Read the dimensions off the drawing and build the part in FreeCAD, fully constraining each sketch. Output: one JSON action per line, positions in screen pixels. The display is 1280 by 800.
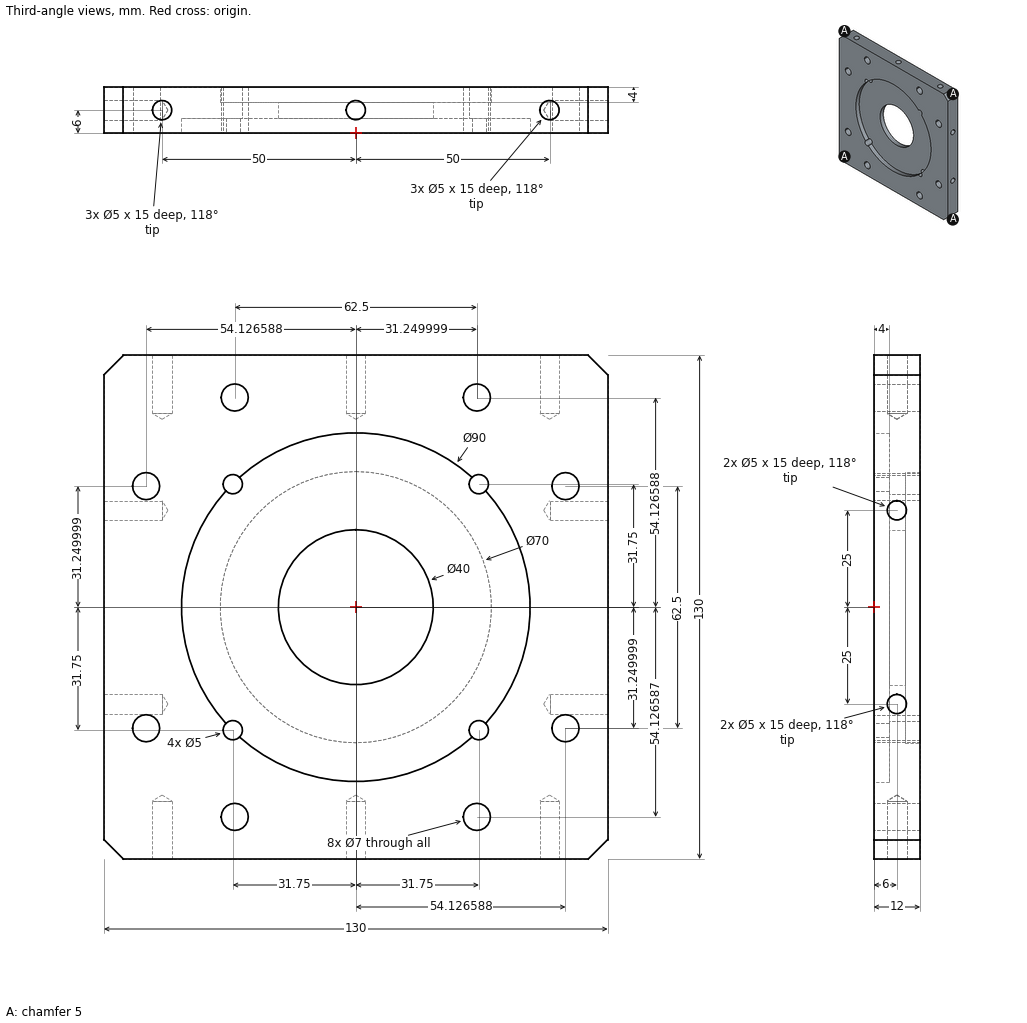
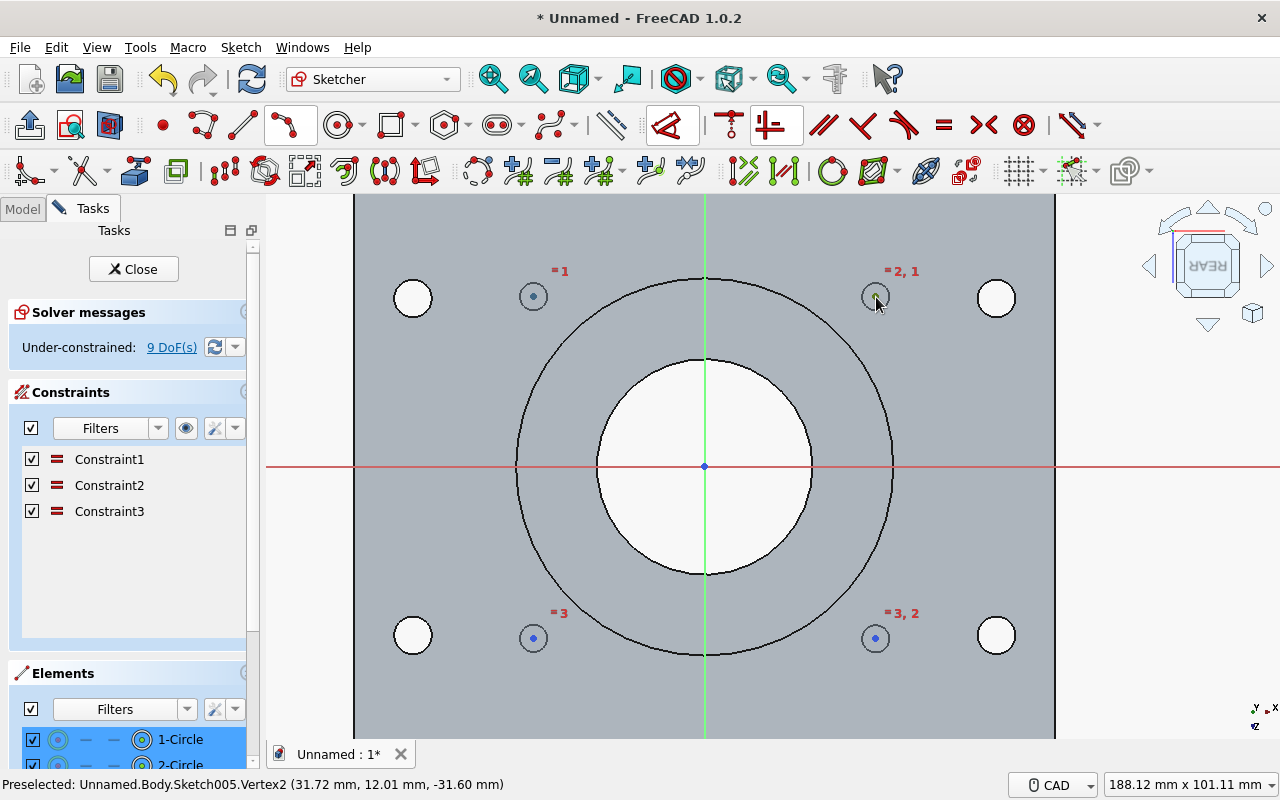
{"action": "left_click", "coordinate": [798, 126]}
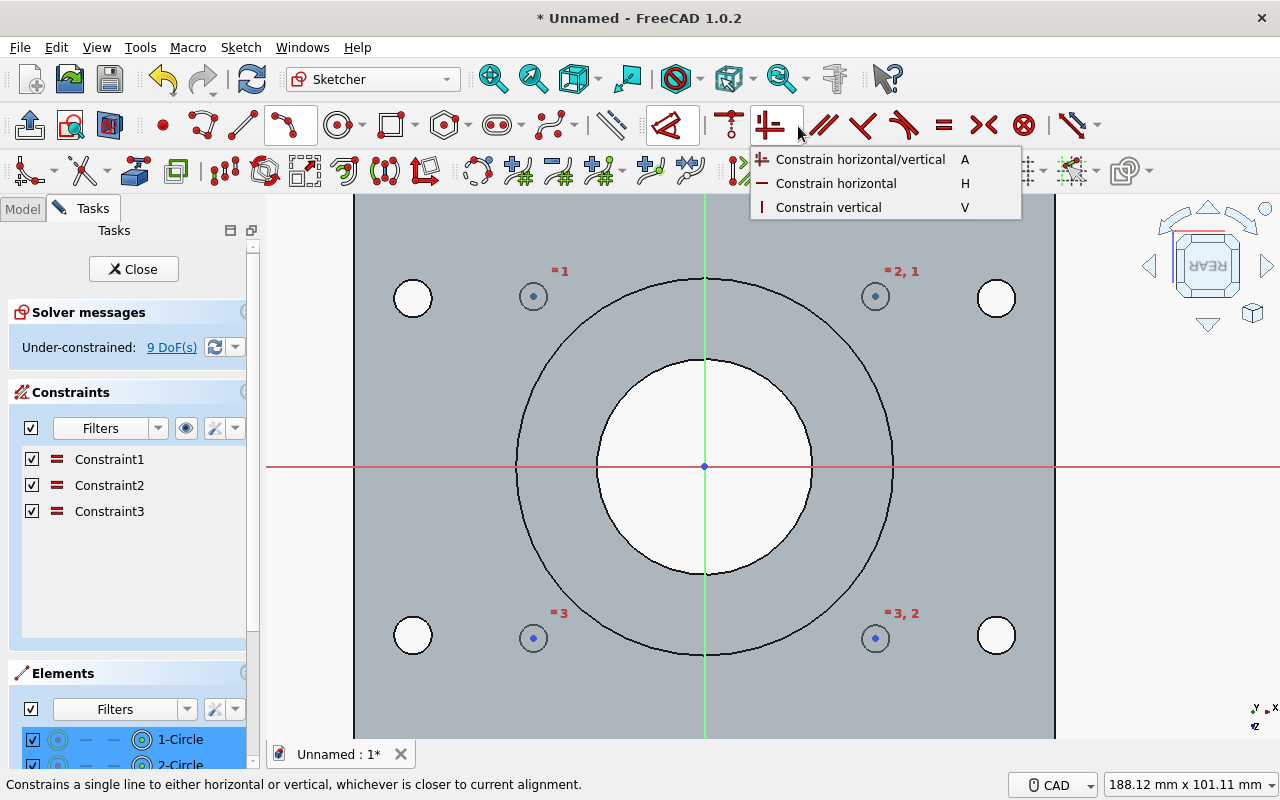
{"action": "left_click", "coordinate": [886, 183]}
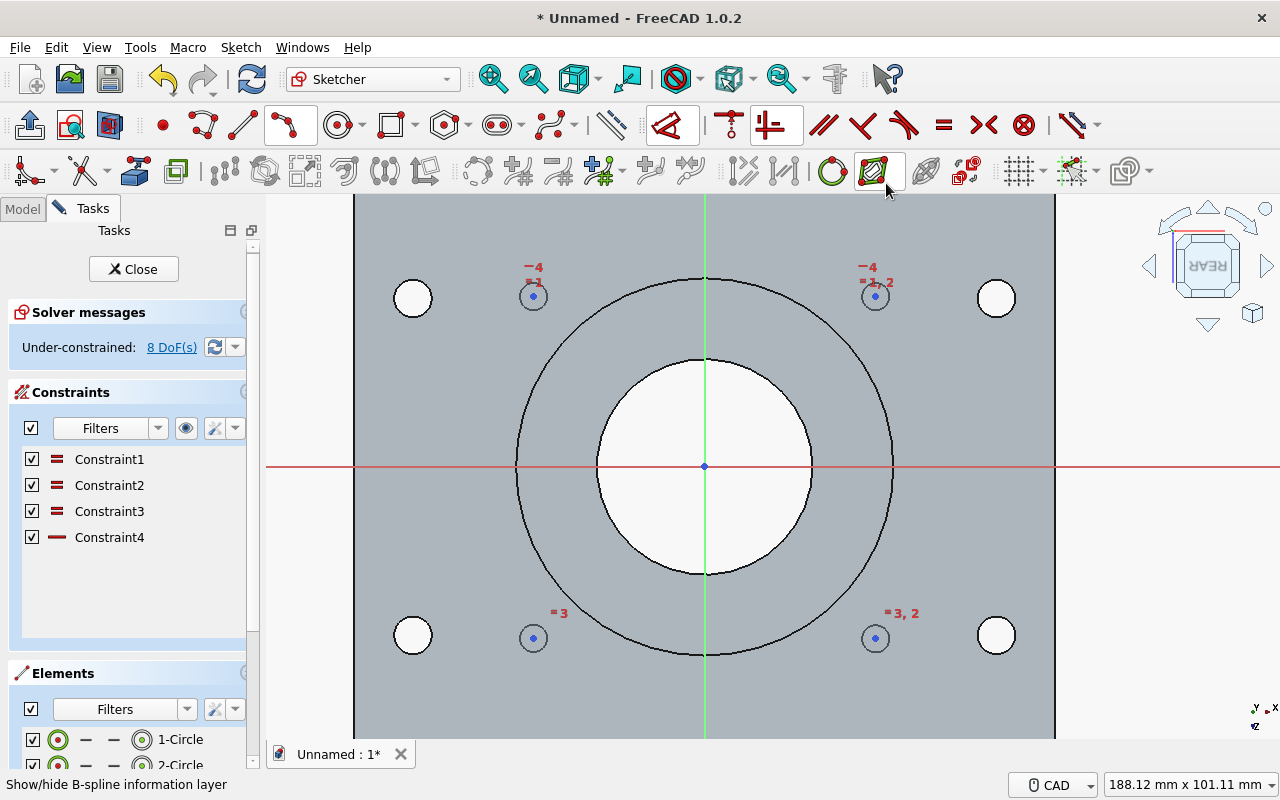
{"action": "left_click", "coordinate": [876, 297]}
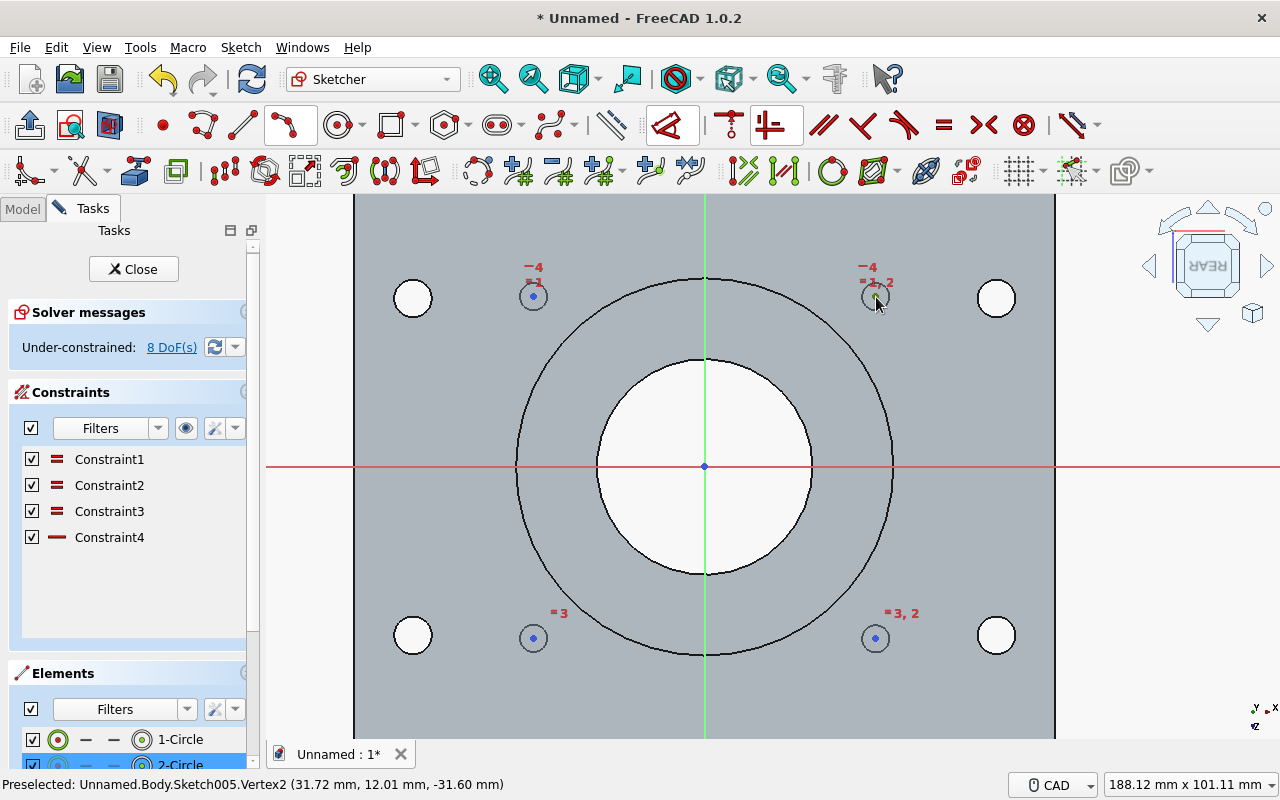
{"action": "left_click", "coordinate": [876, 639]}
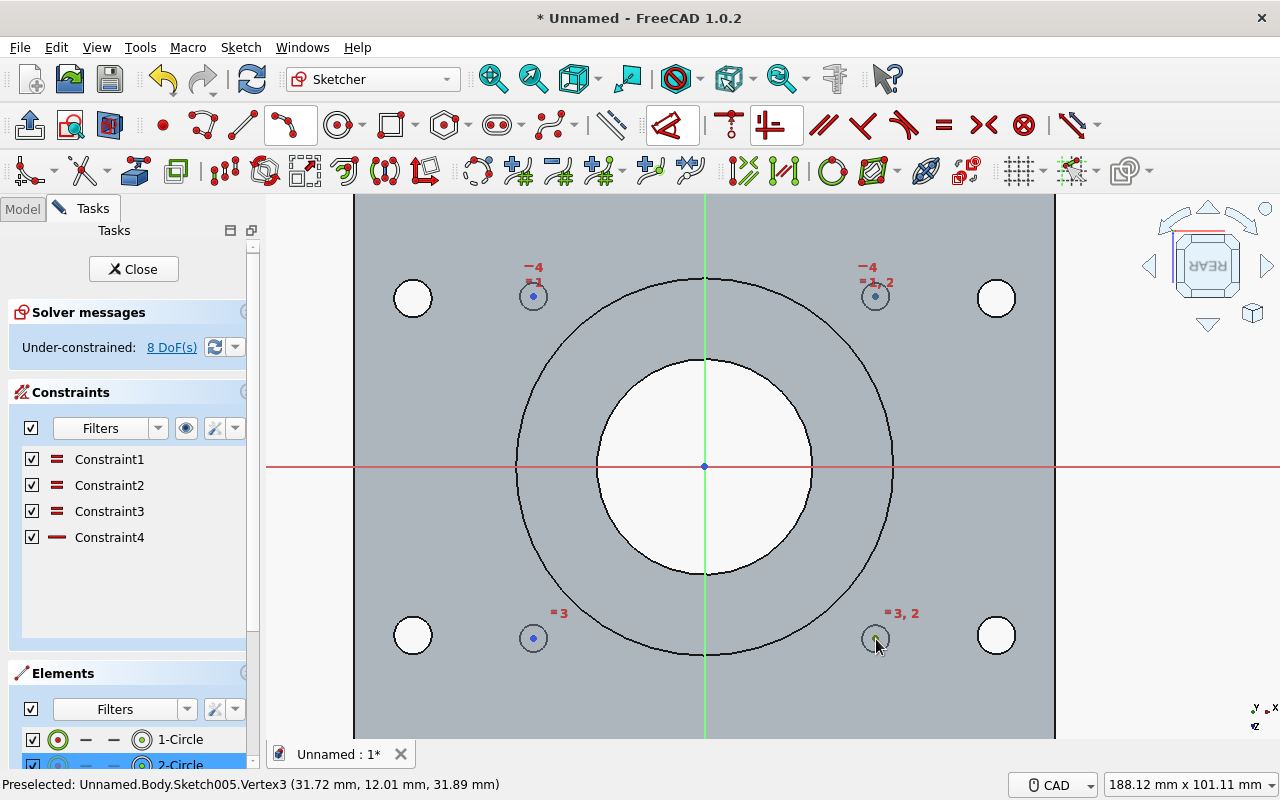
{"action": "left_click", "coordinate": [798, 126]}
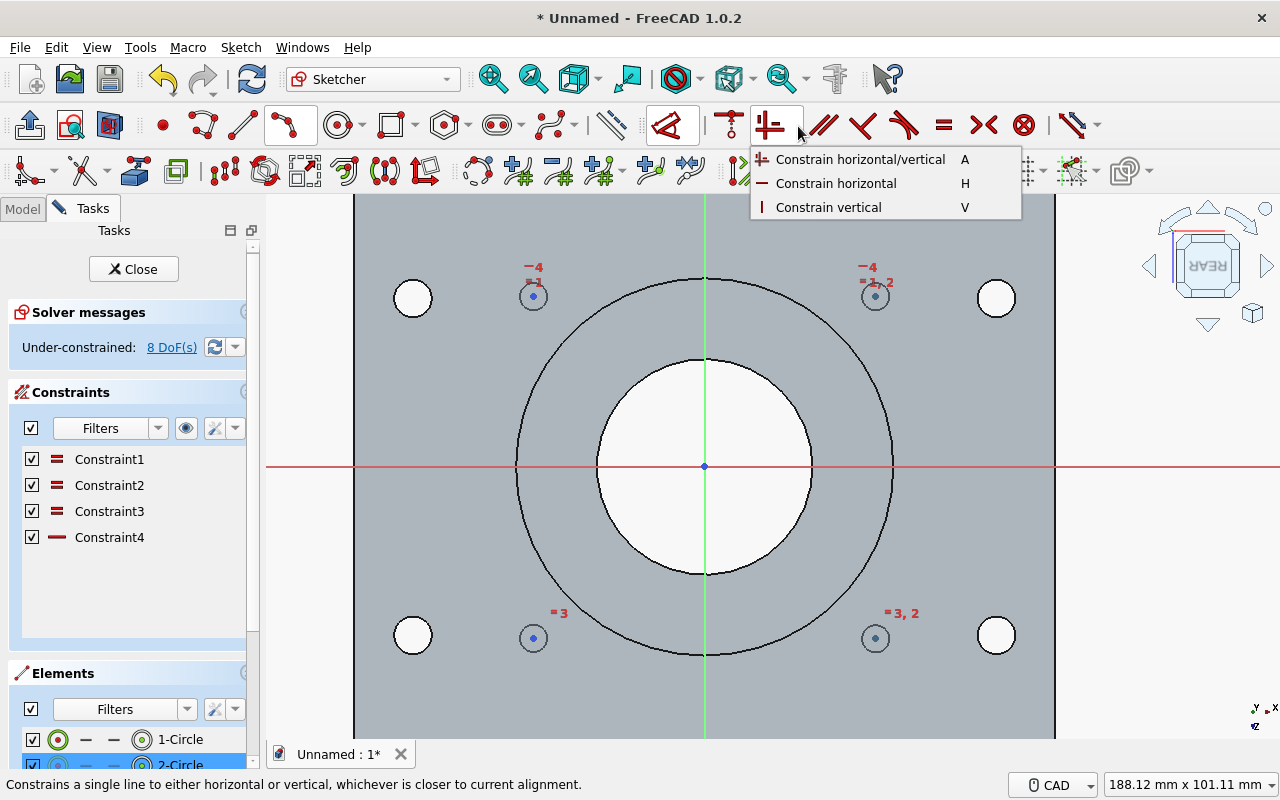
{"action": "left_click", "coordinate": [886, 207]}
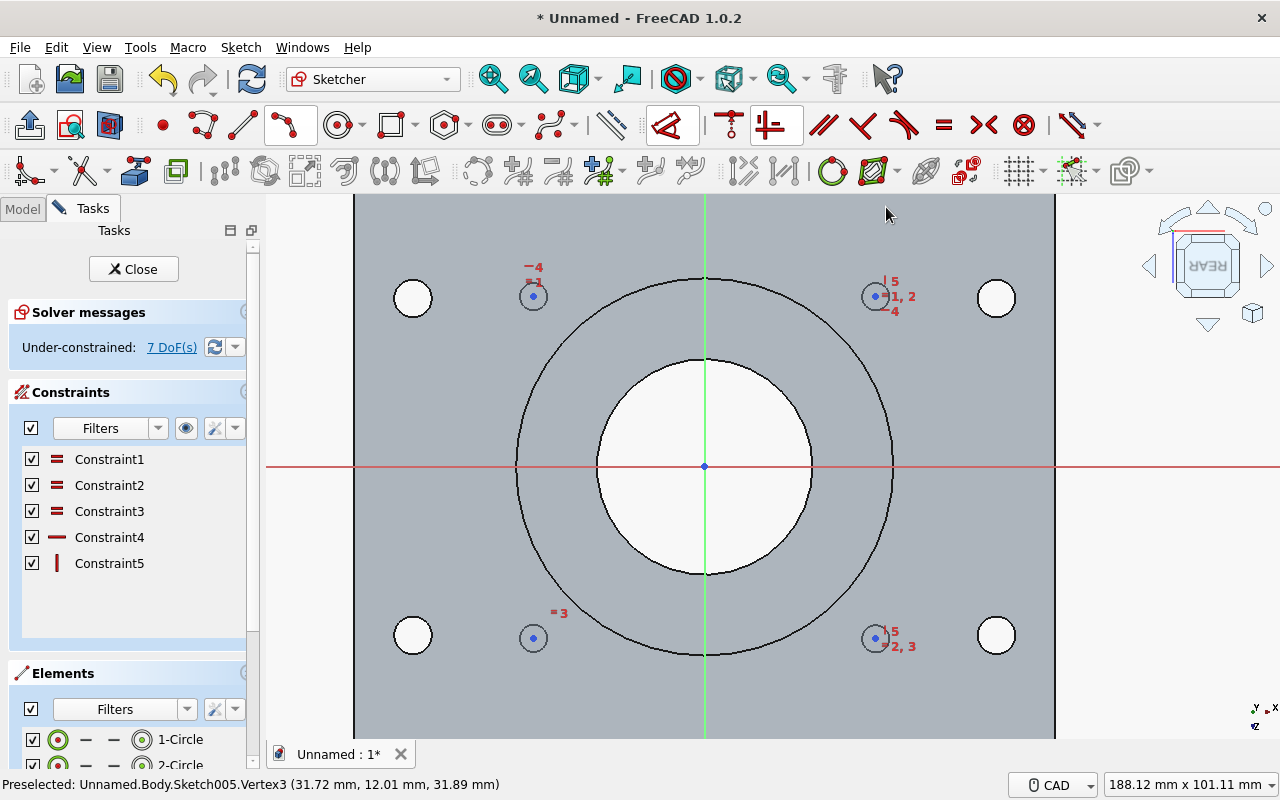
{"action": "left_click", "coordinate": [534, 297]}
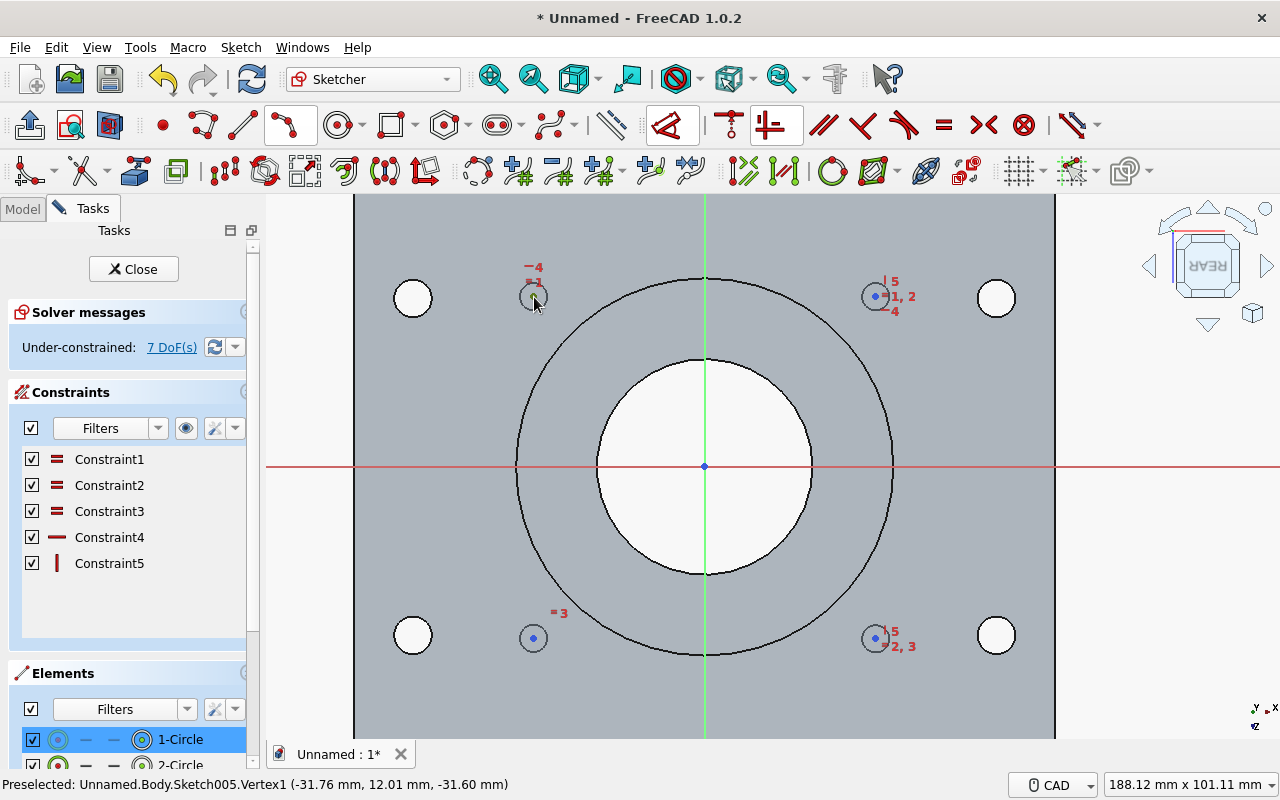
{"action": "left_click", "coordinate": [534, 638]}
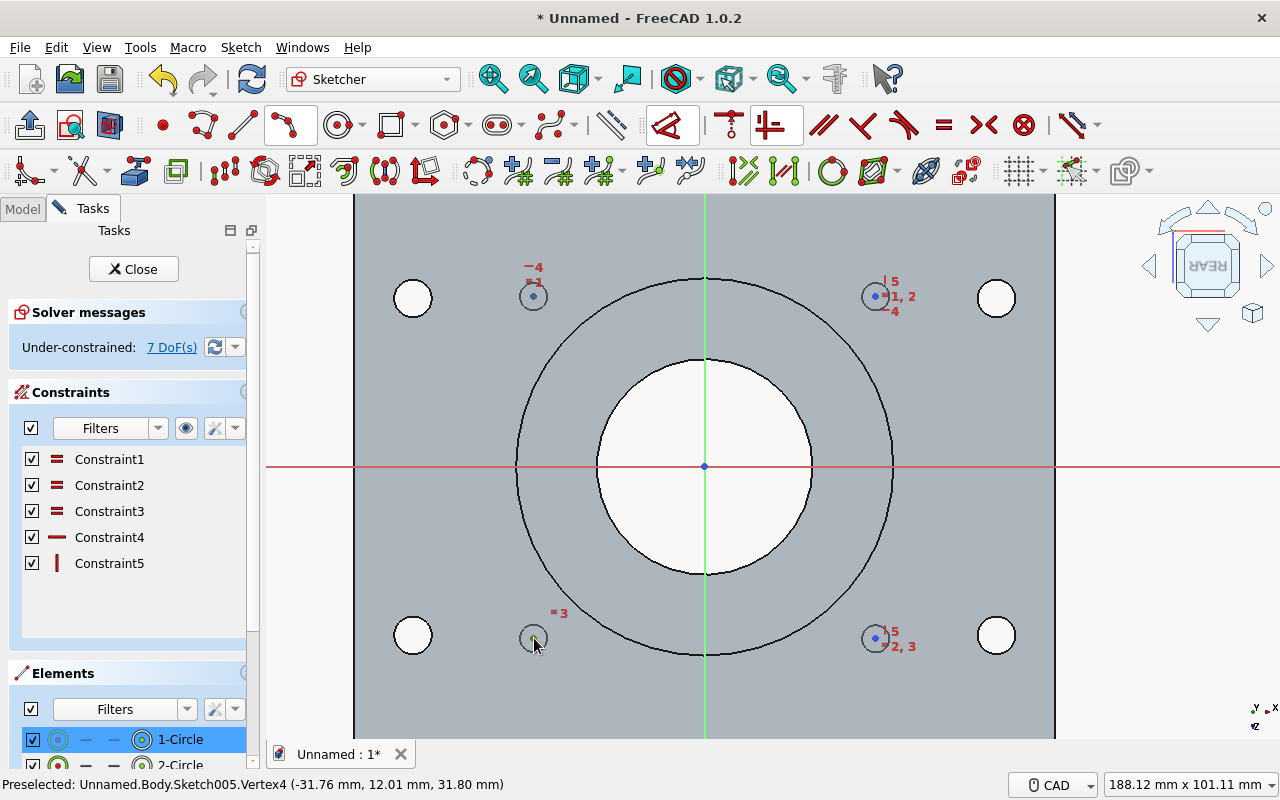
{"action": "left_click", "coordinate": [798, 126]}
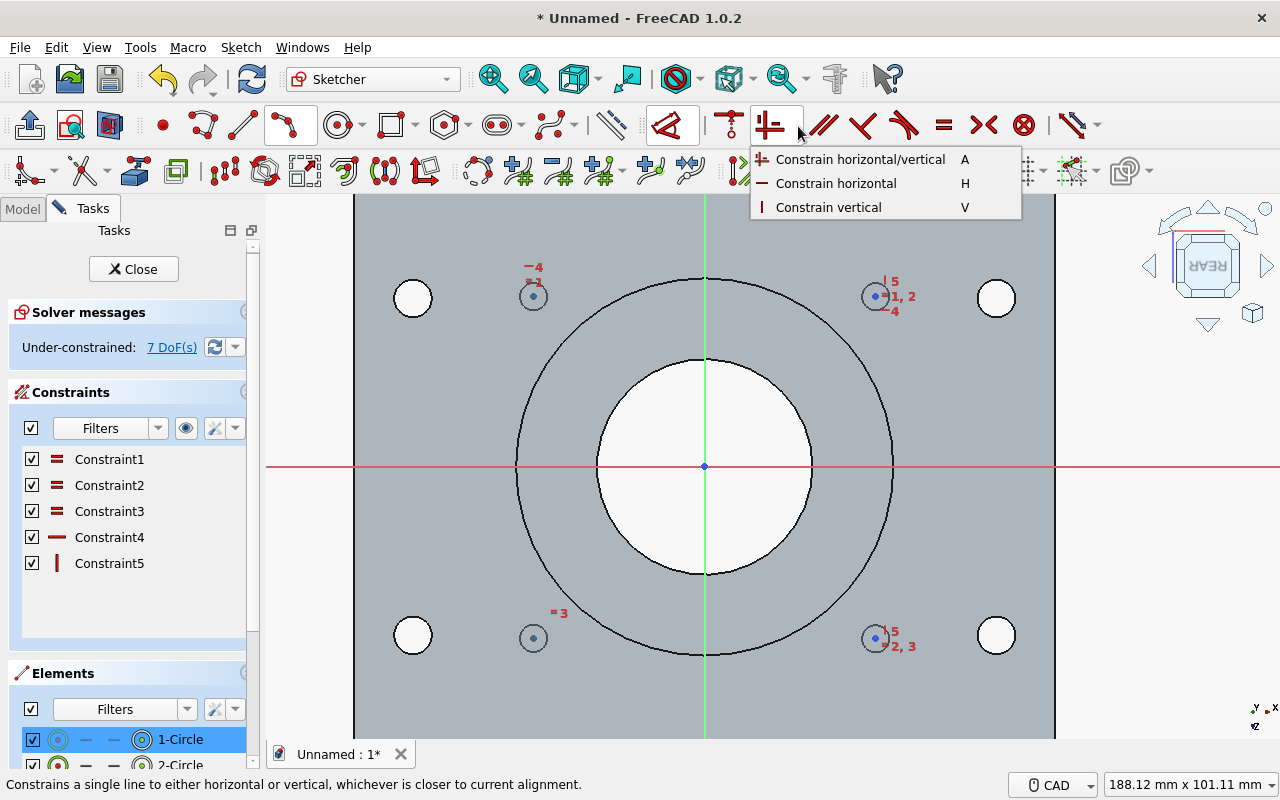
{"action": "left_click", "coordinate": [886, 207]}